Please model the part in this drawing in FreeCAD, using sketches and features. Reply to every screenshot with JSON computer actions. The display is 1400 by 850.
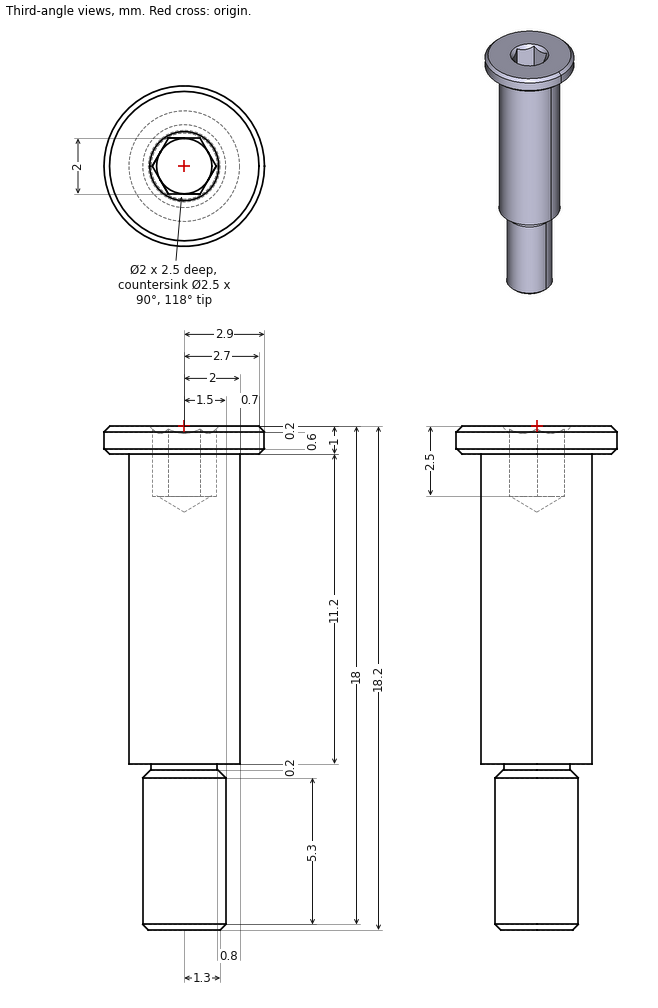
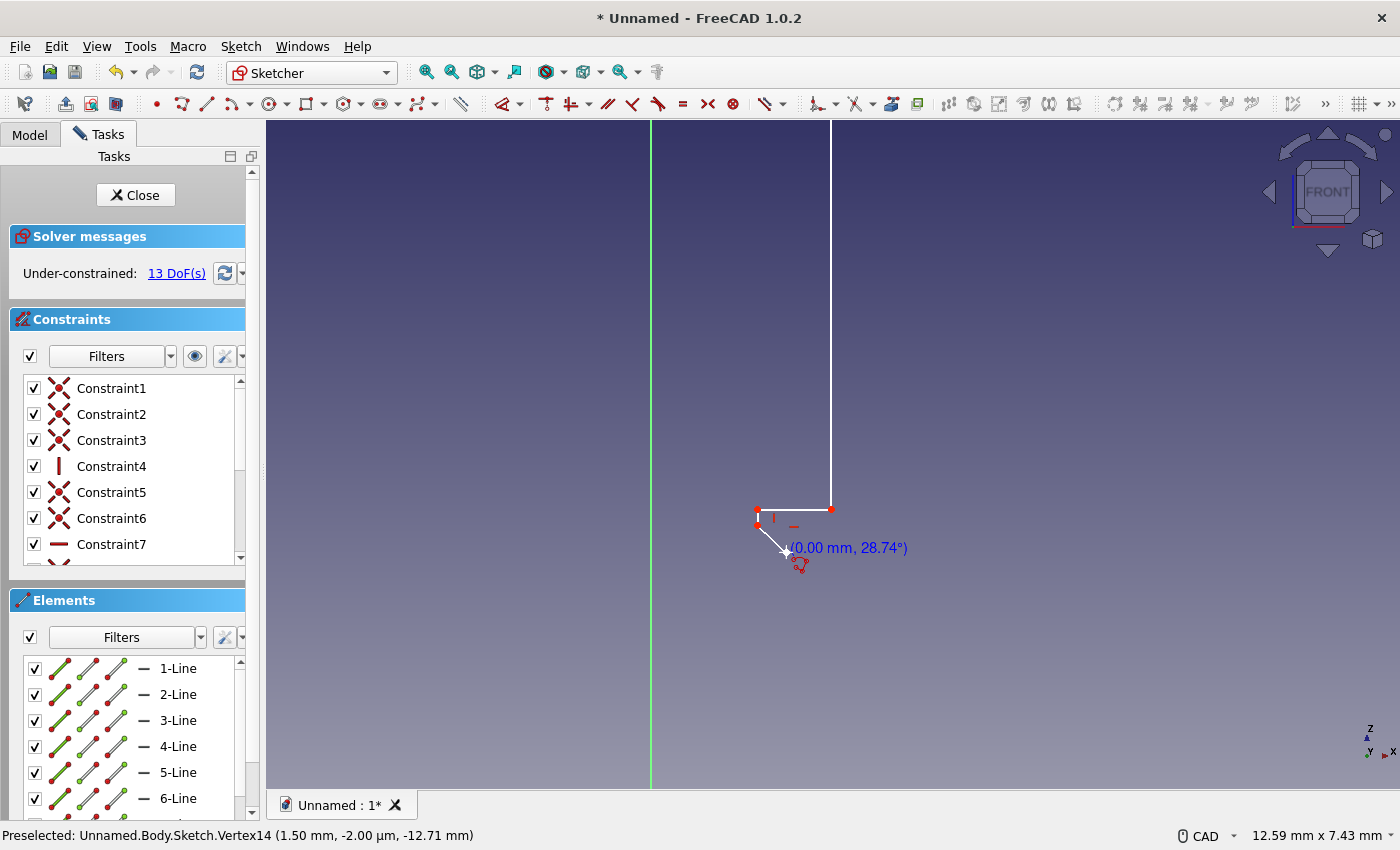
{"action": "scroll", "coordinate": [759, 529], "scroll_direction": "down", "scroll_amount": 7}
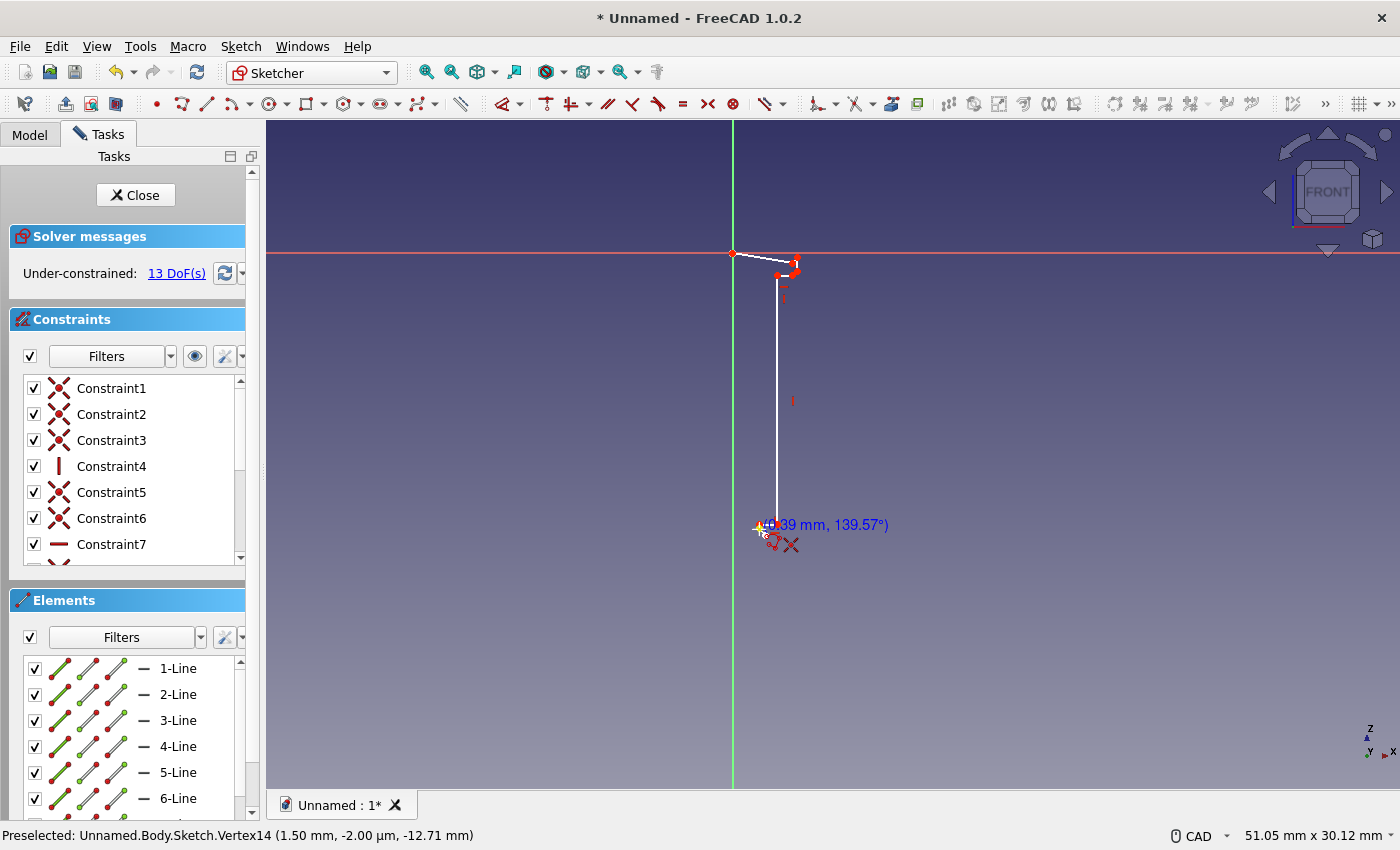
{"action": "left_click", "coordinate": [766, 653]}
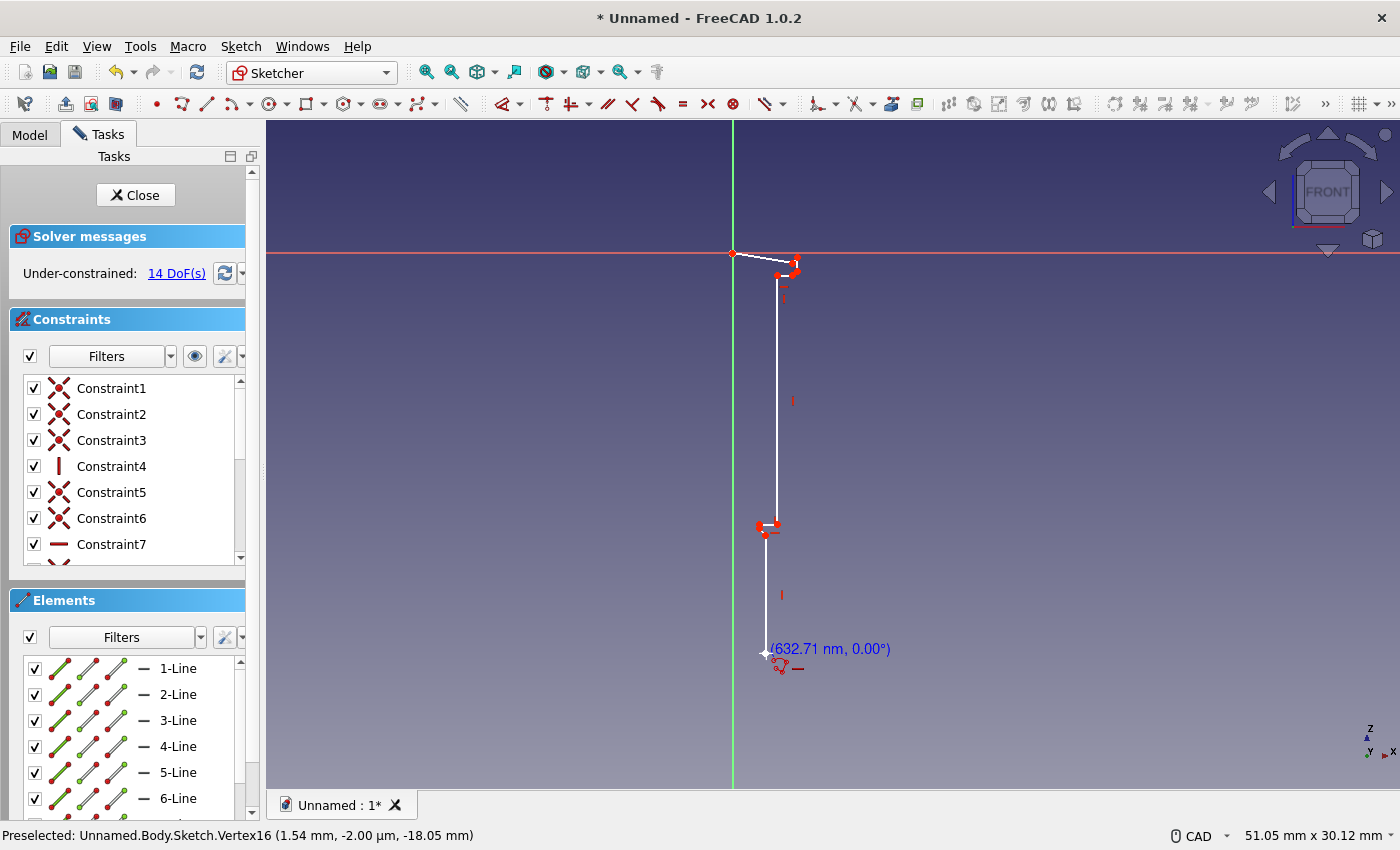
{"action": "scroll", "coordinate": [762, 657], "scroll_direction": "up", "scroll_amount": 5}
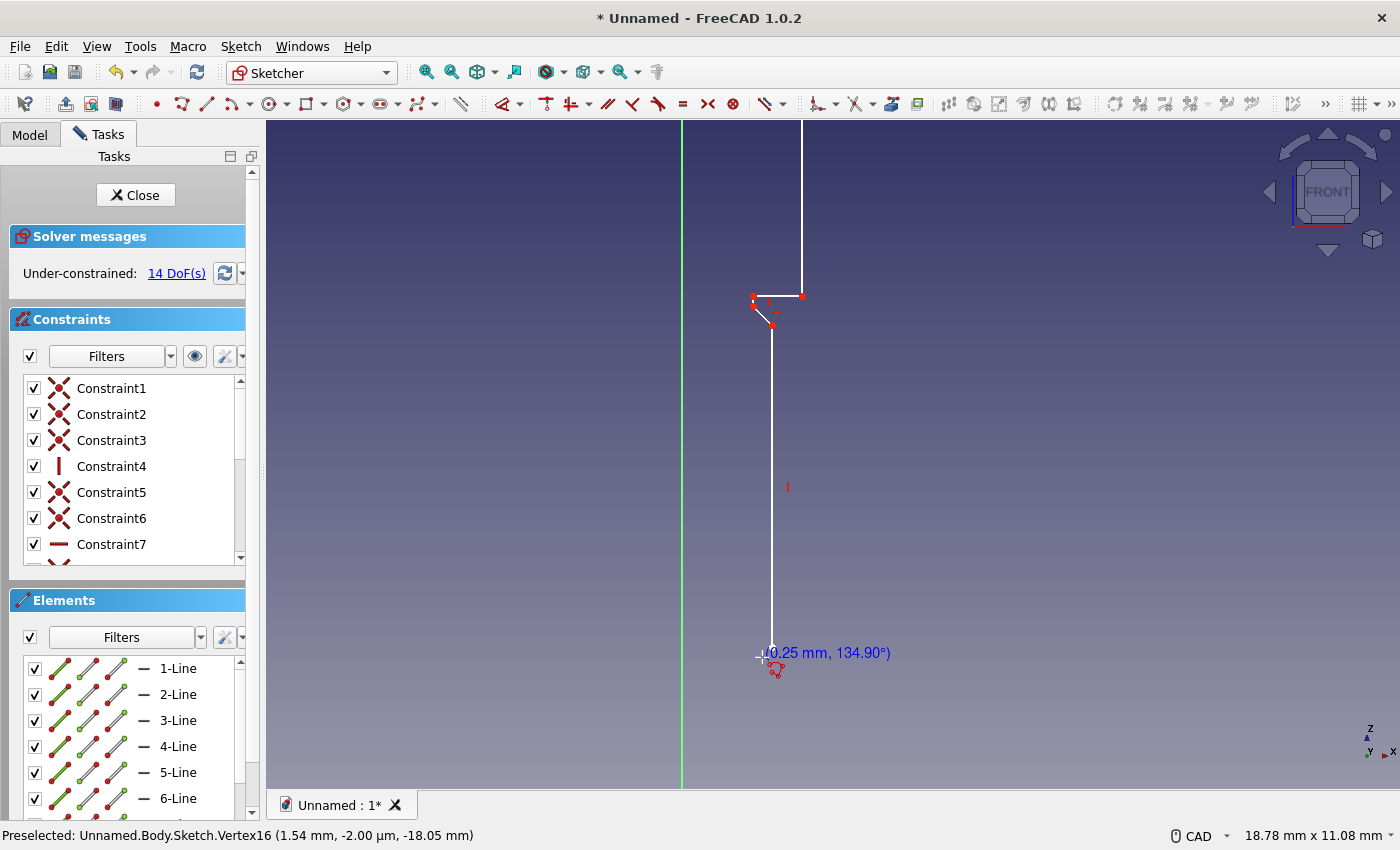
{"action": "left_click", "coordinate": [760, 656]}
{"action": "left_click", "coordinate": [691, 656]}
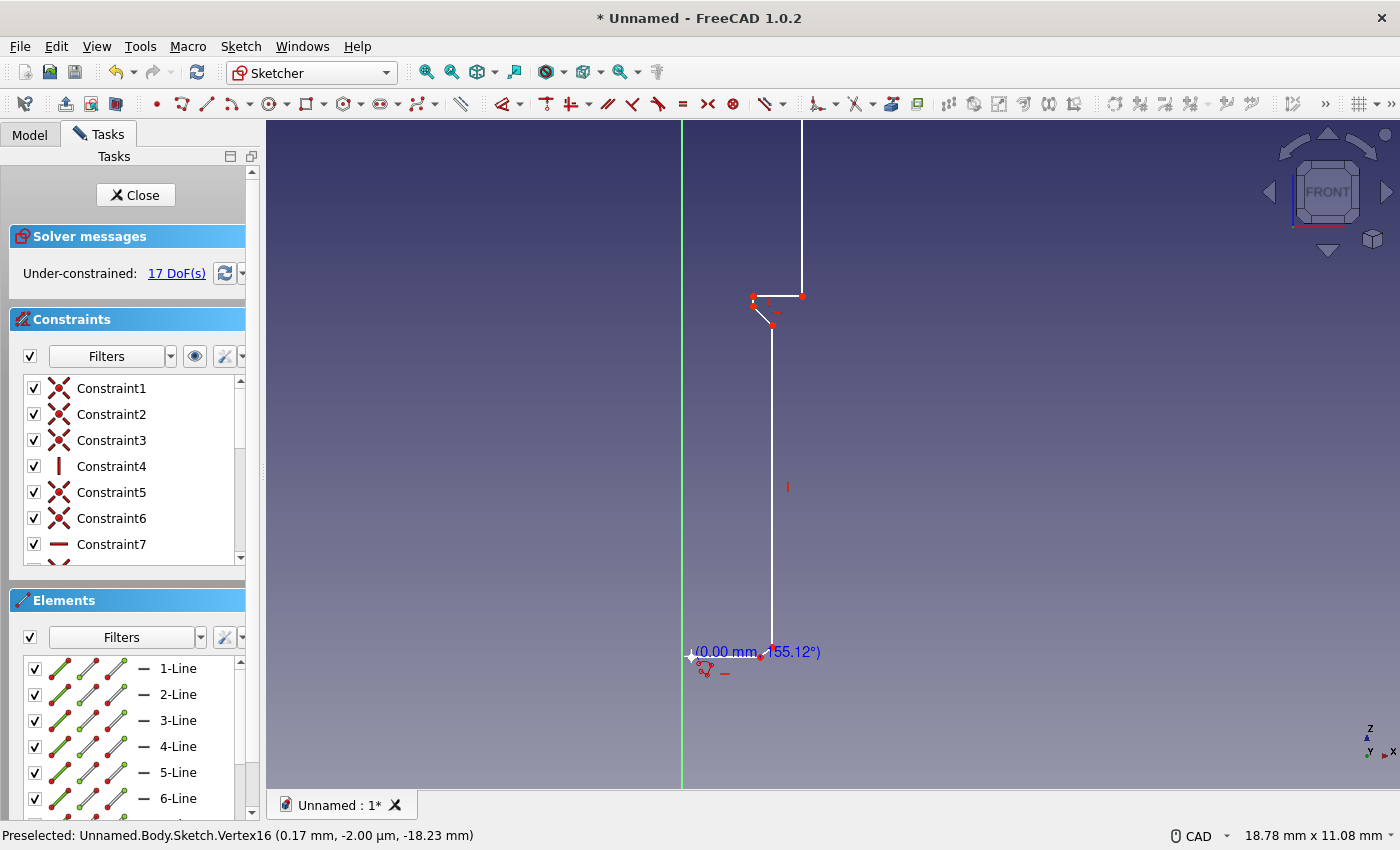
{"action": "scroll", "coordinate": [762, 657], "scroll_direction": "down", "scroll_amount": 5}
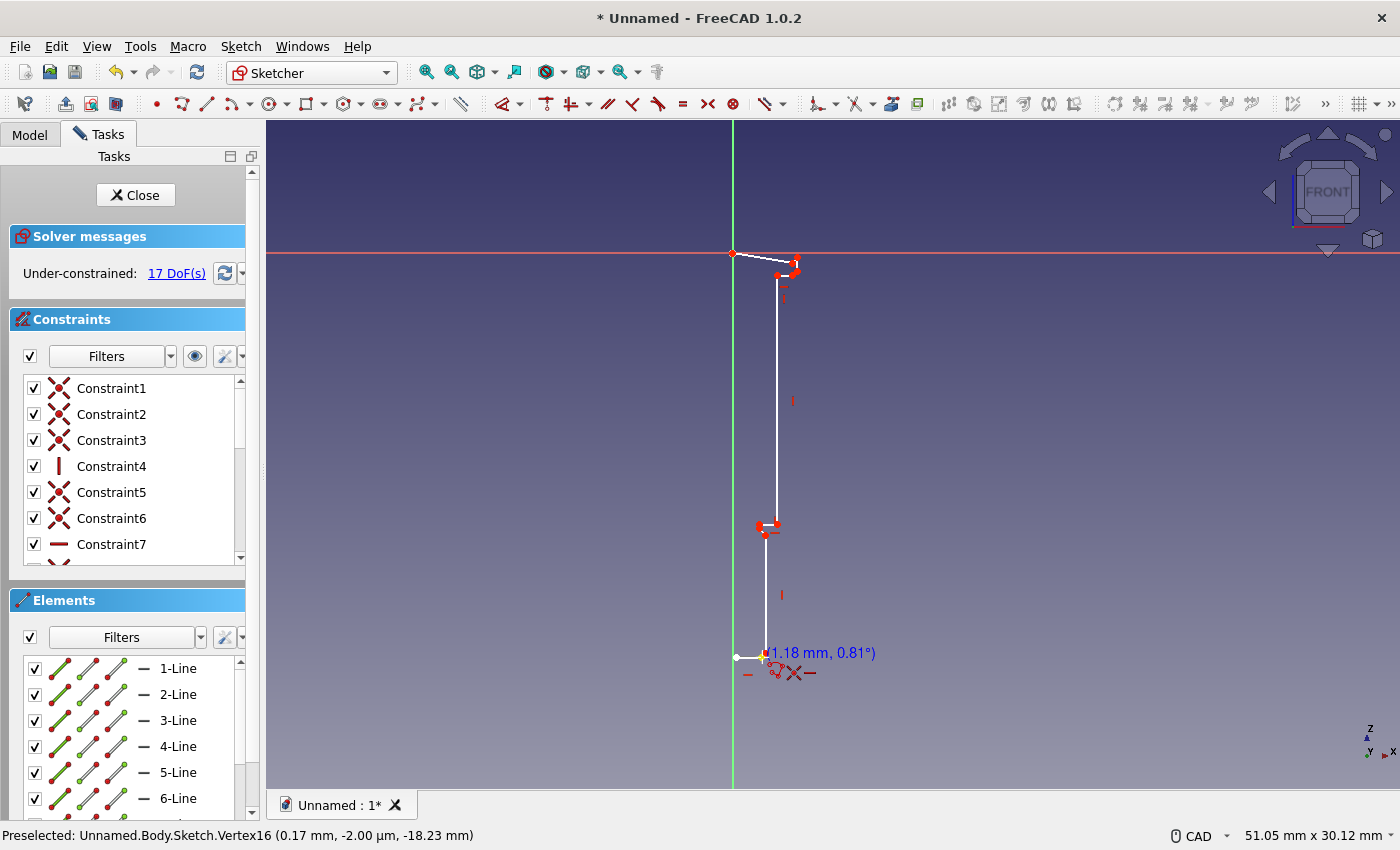
{"action": "left_click", "coordinate": [733, 253]}
{"action": "key", "text": "Escape"}
{"action": "key", "text": "Escape"}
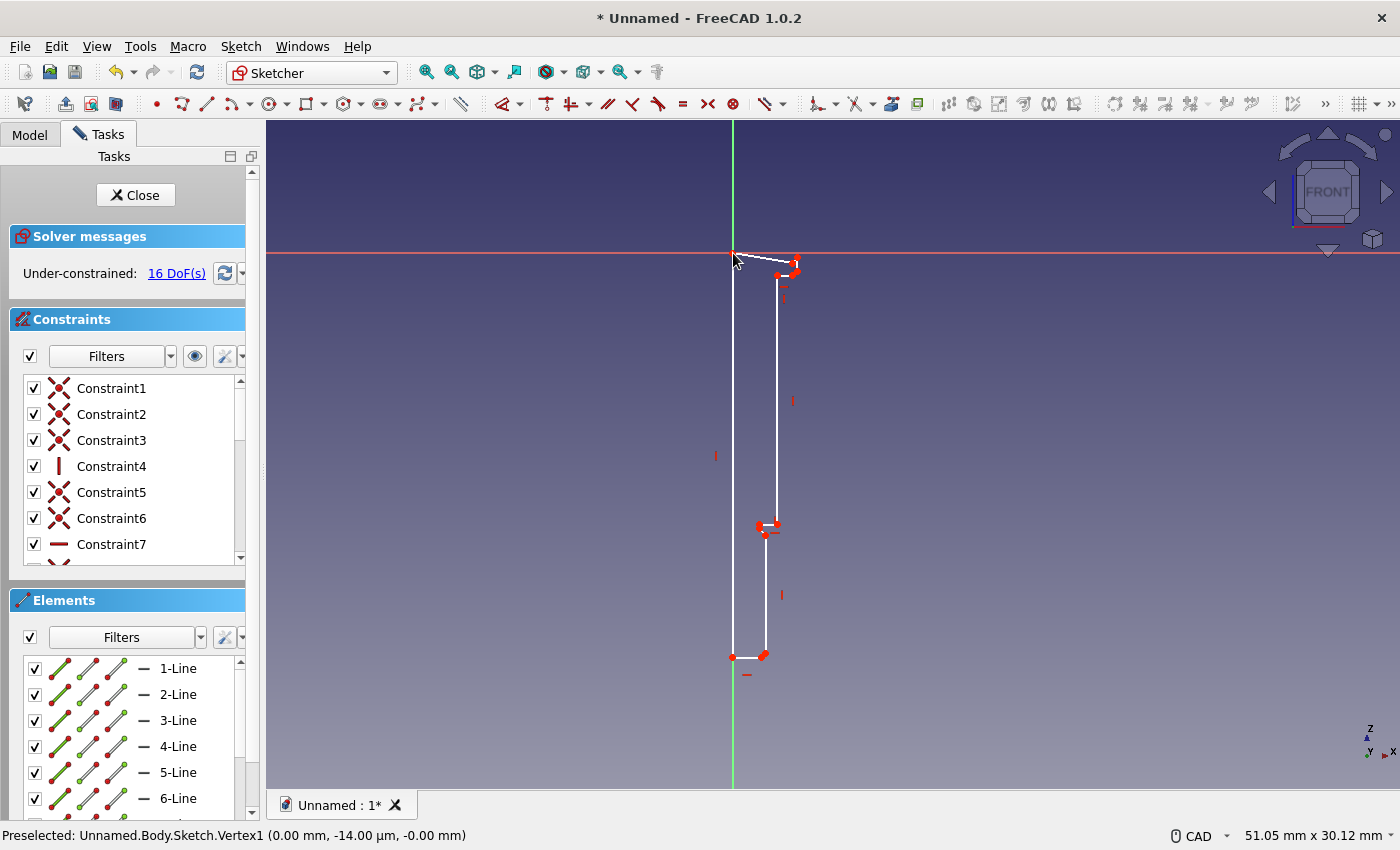
{"action": "left_click", "coordinate": [751, 256]}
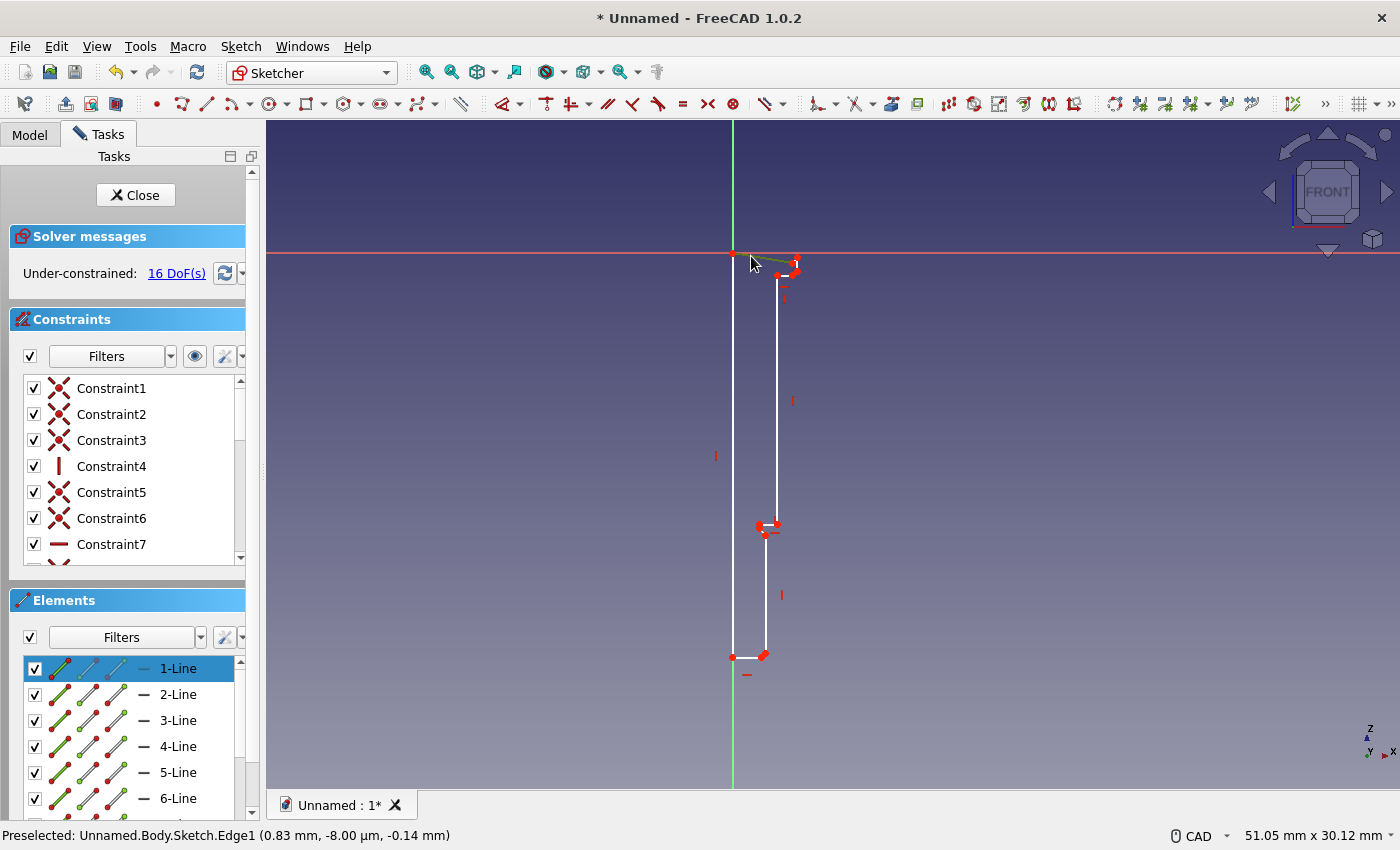
{"action": "key", "text": "h"}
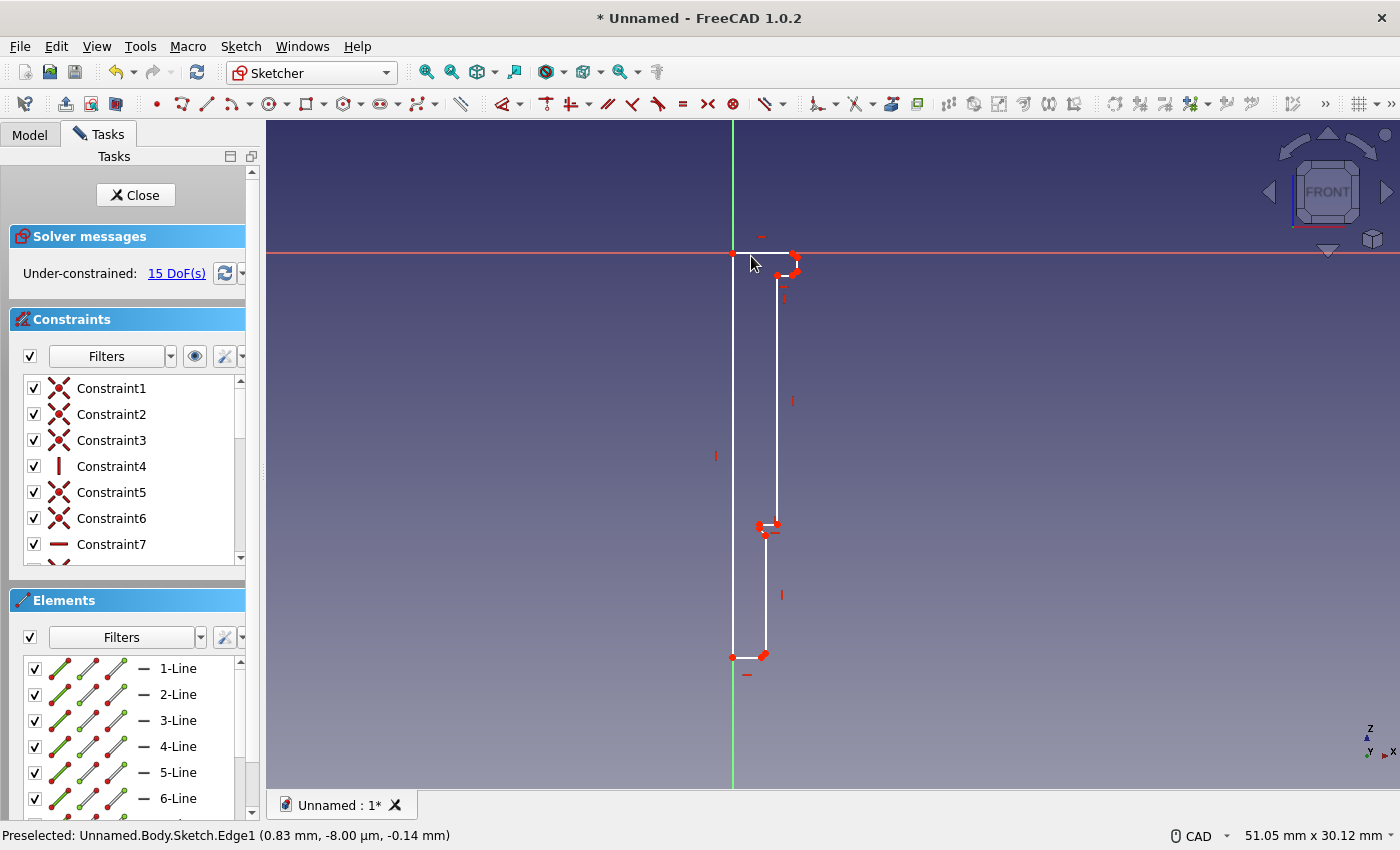
{"action": "left_click", "coordinate": [502, 104]}